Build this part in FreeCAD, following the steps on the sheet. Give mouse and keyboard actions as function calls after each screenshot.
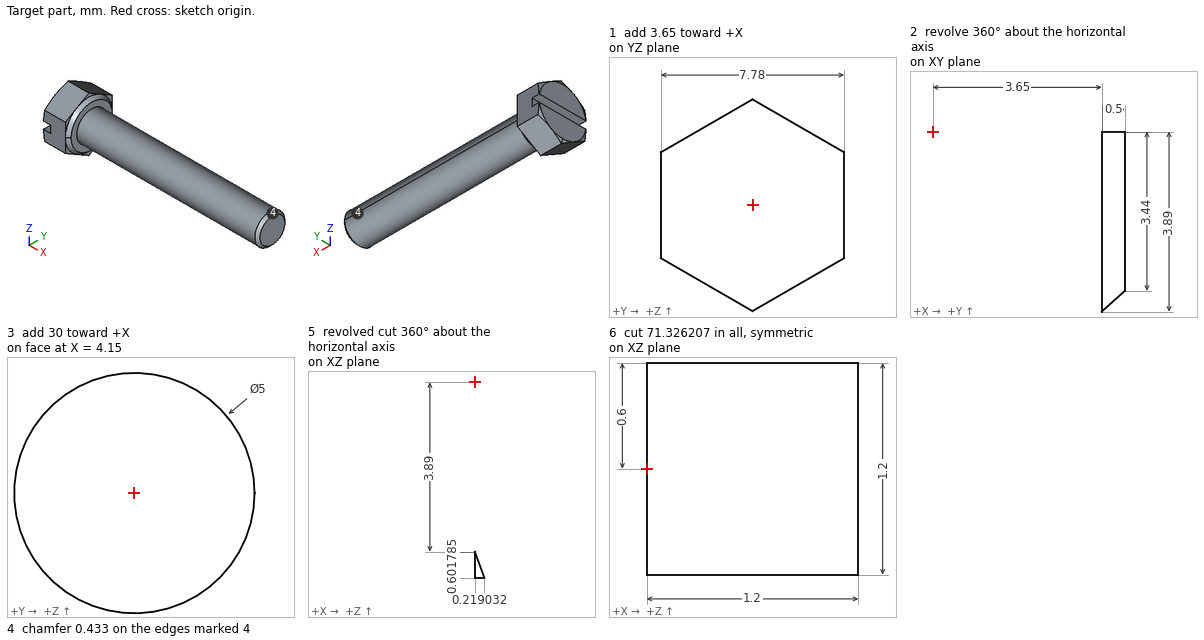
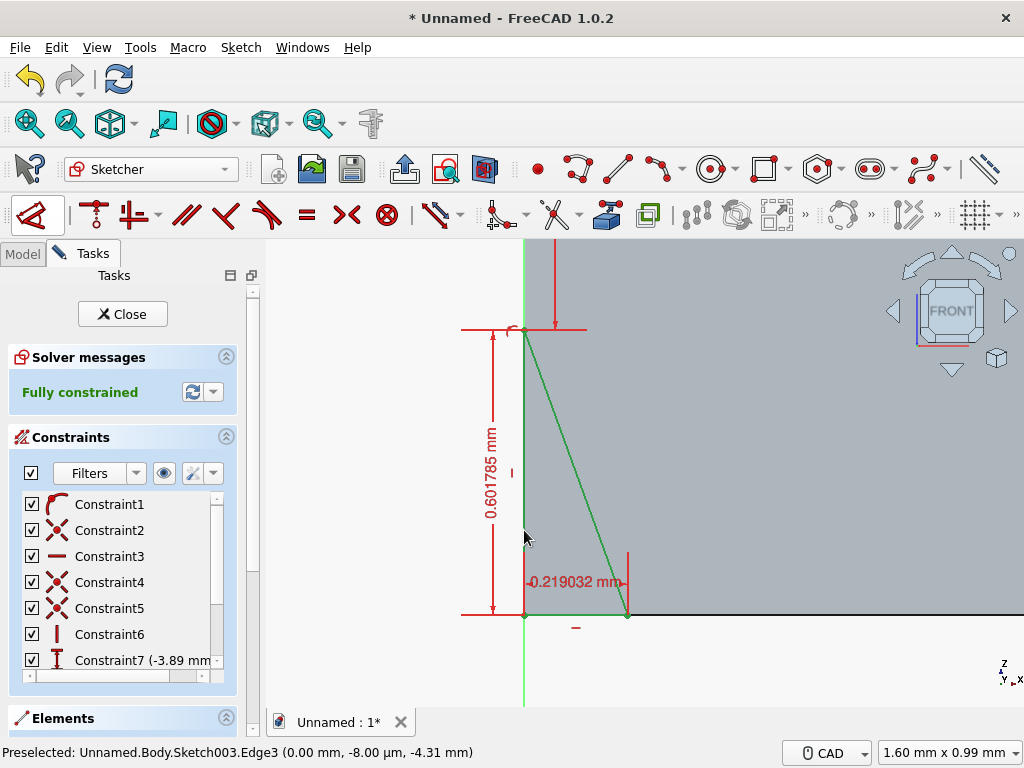
click(123, 314)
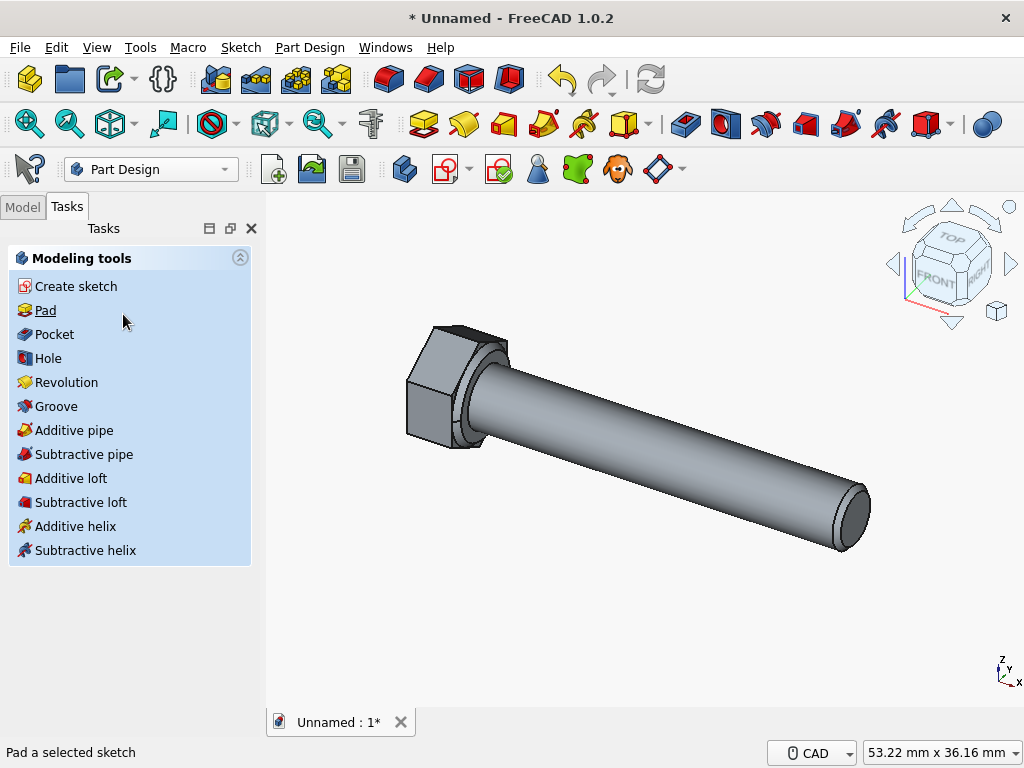
click(766, 124)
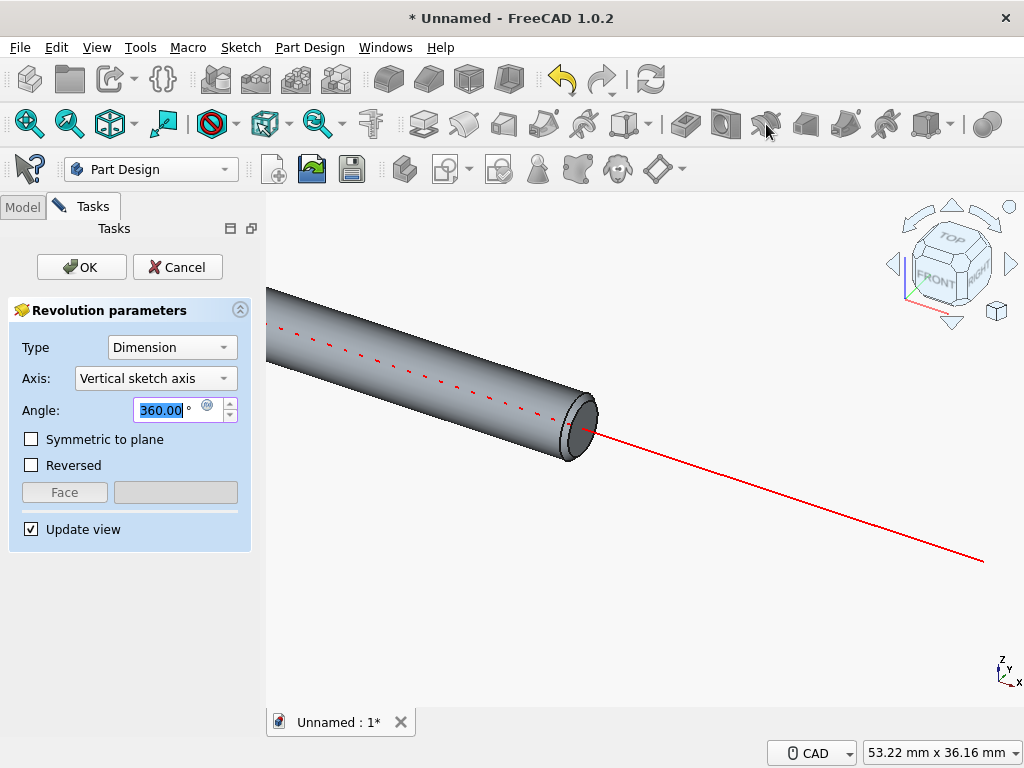
click(156, 378)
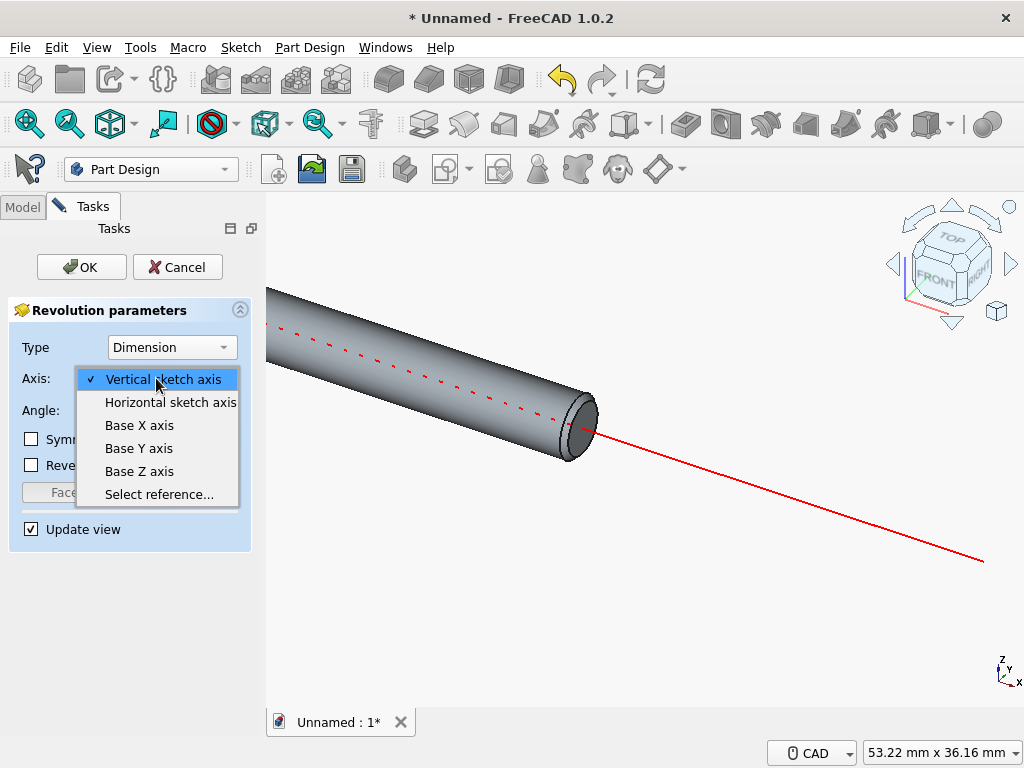
click(156, 402)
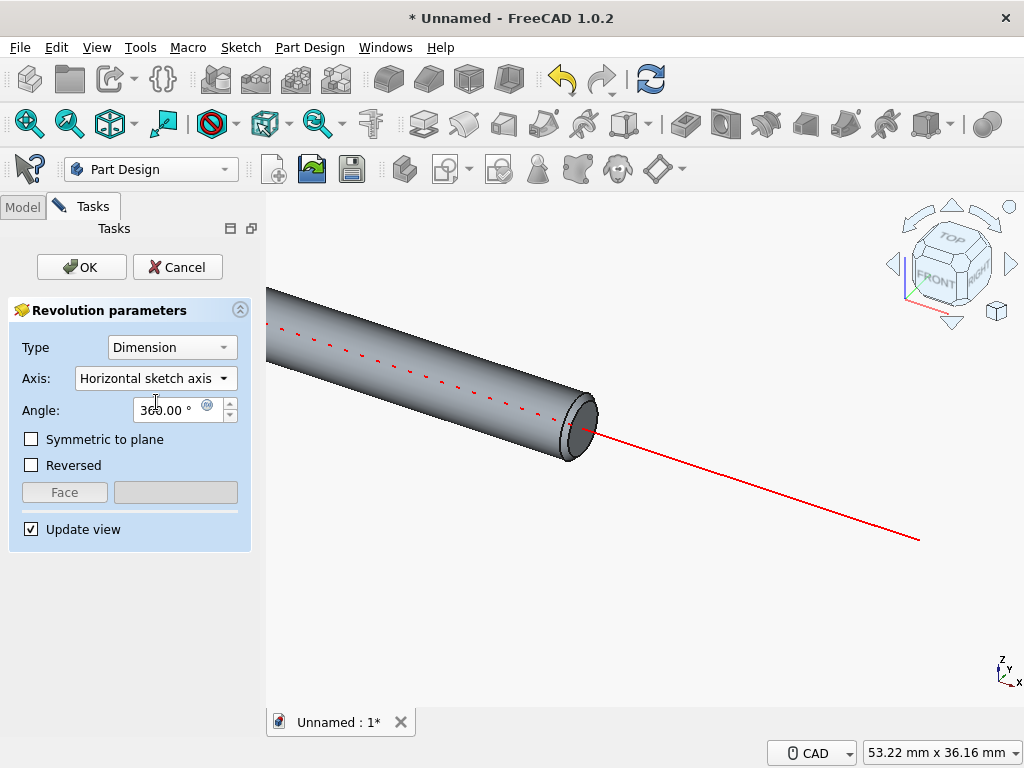
click(82, 267)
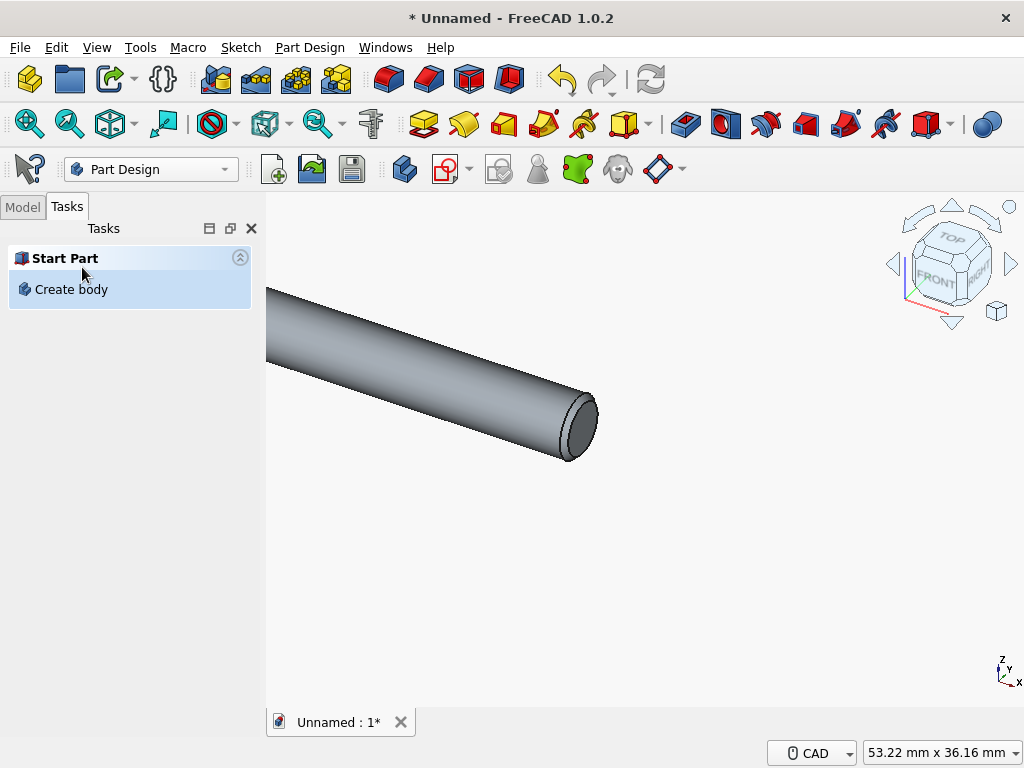
click(30, 124)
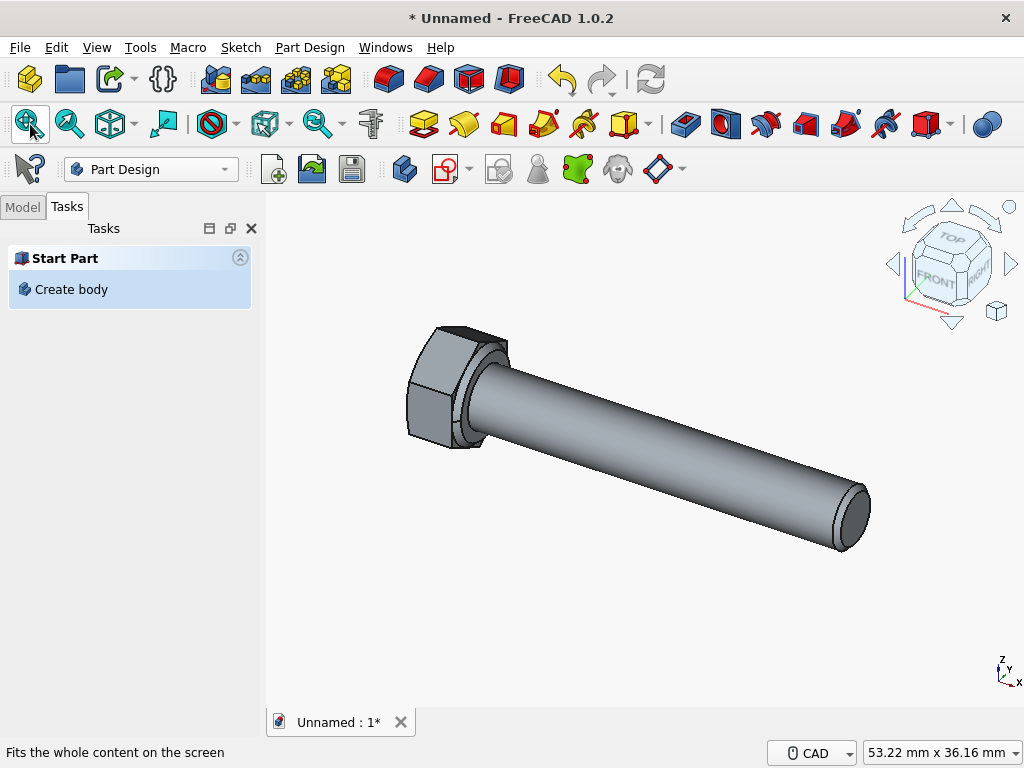
click(446, 170)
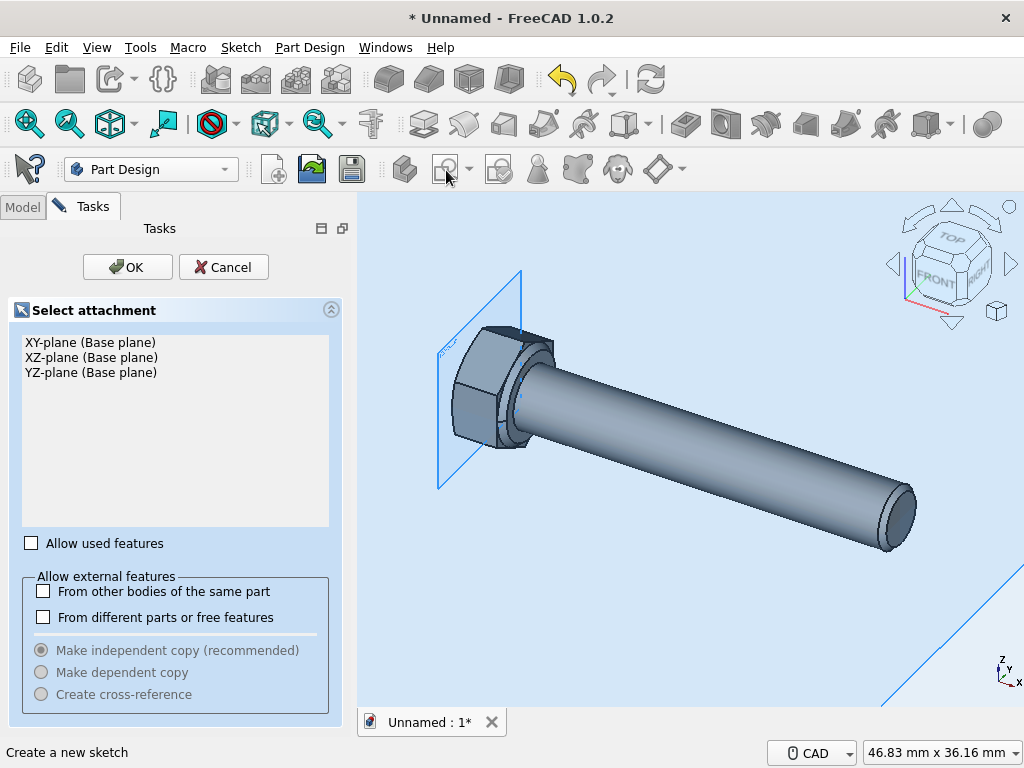
click(82, 358)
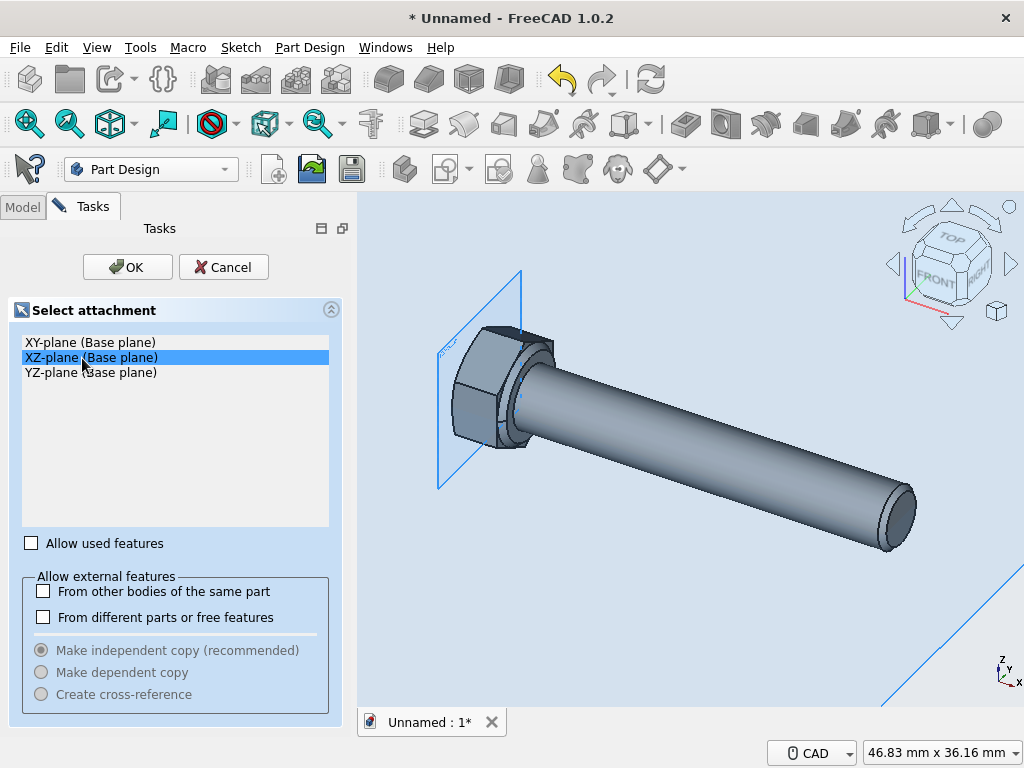
click(128, 267)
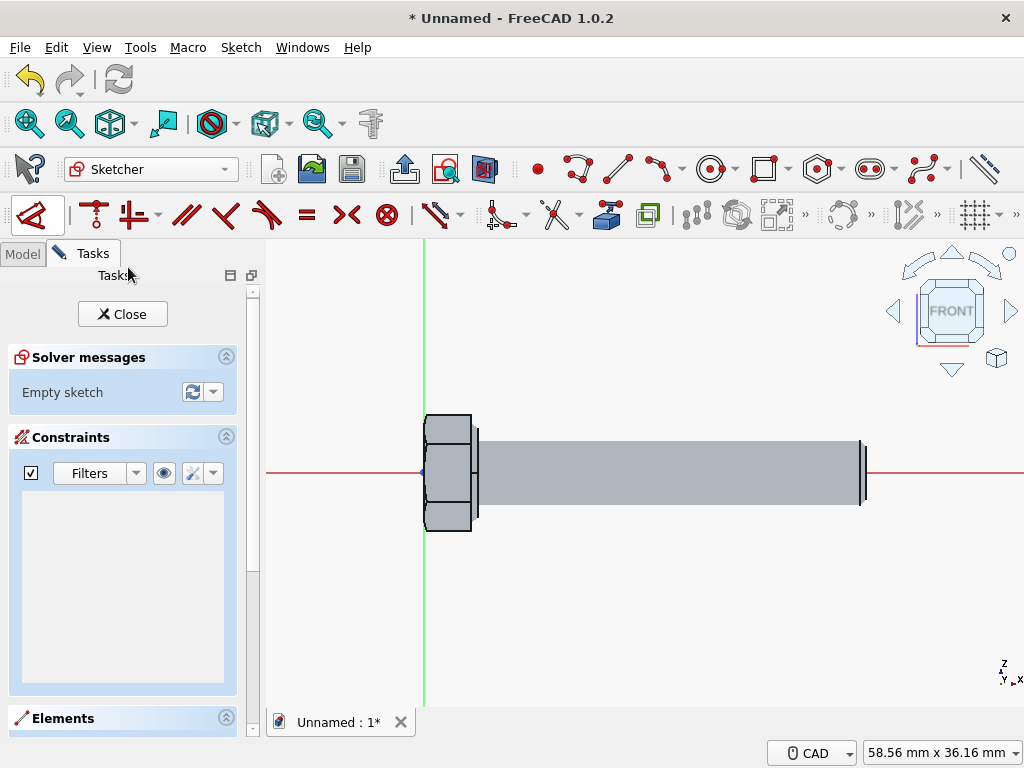
key(q)
key(s)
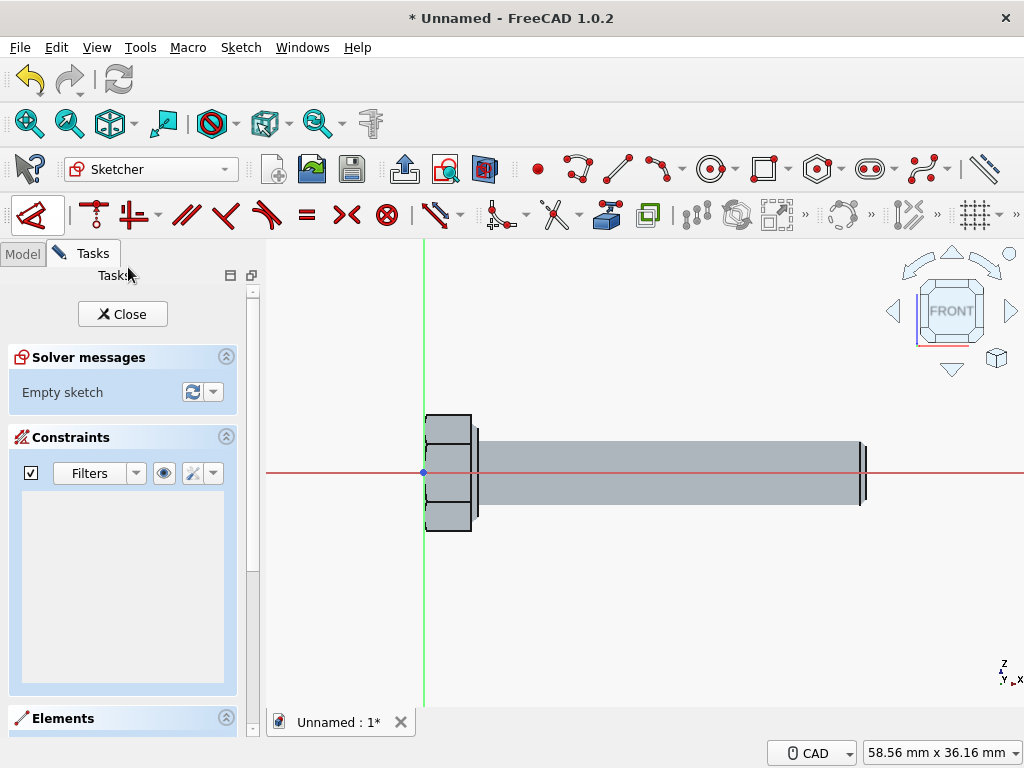
scroll(424, 473, up, 15)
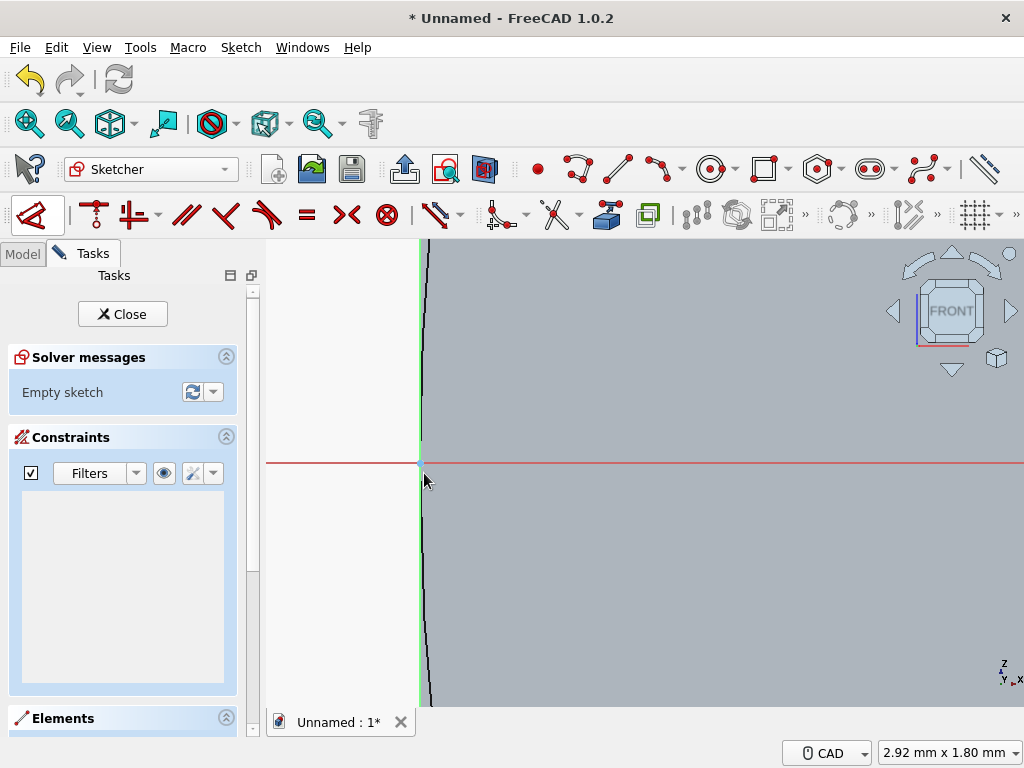
key(g)
key(r)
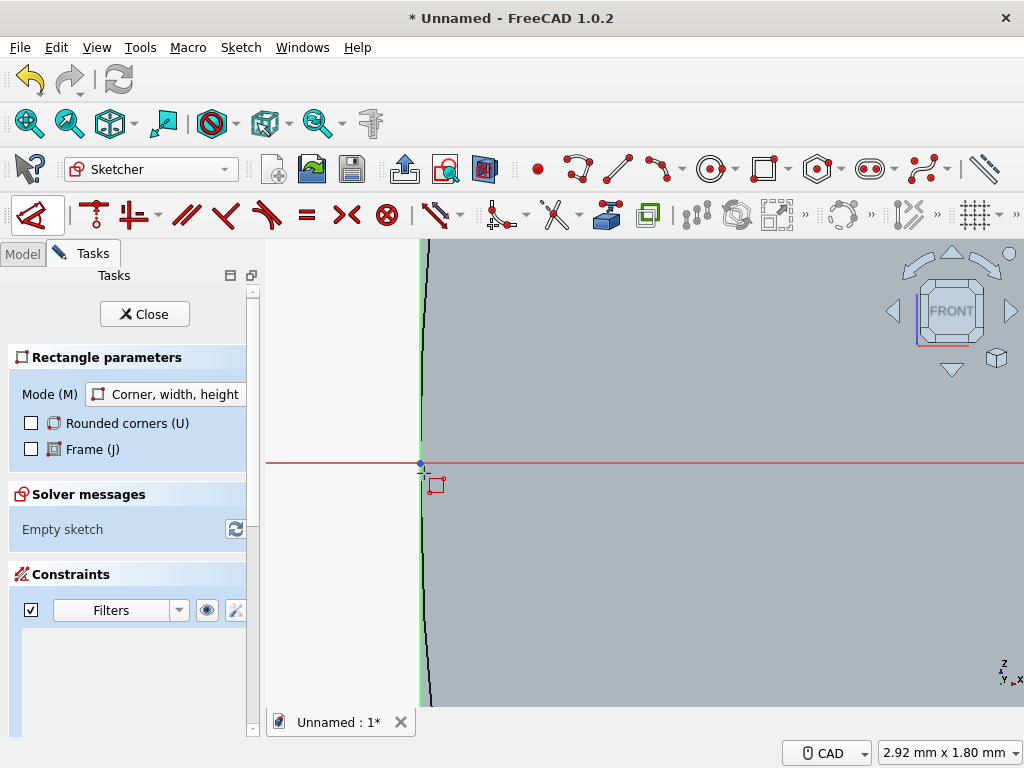
click(420, 307)
move(732, 619)